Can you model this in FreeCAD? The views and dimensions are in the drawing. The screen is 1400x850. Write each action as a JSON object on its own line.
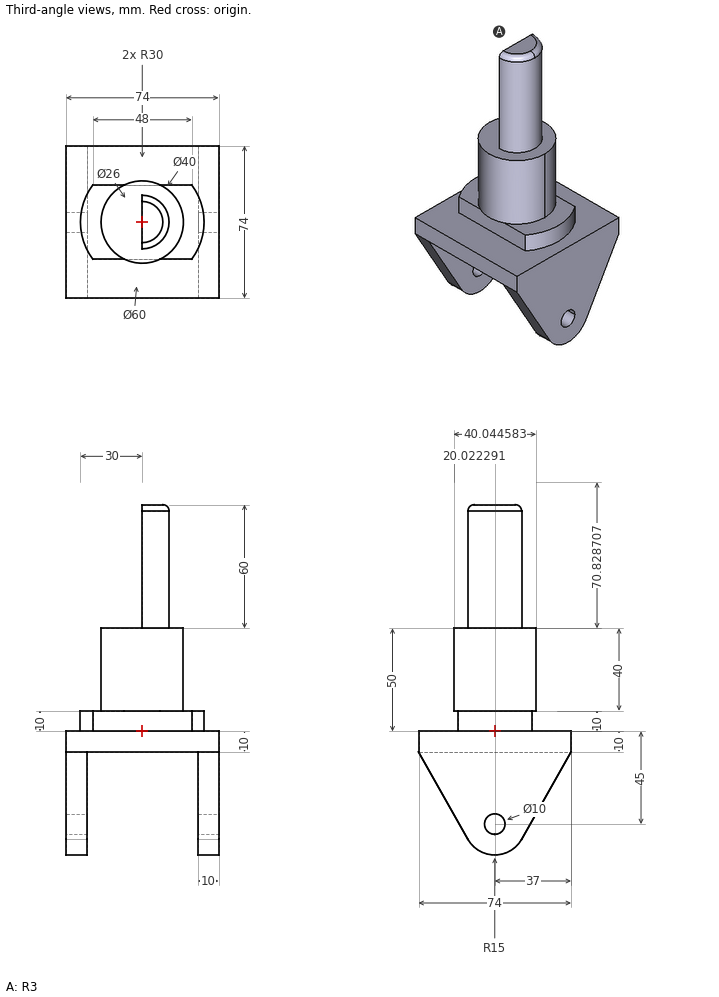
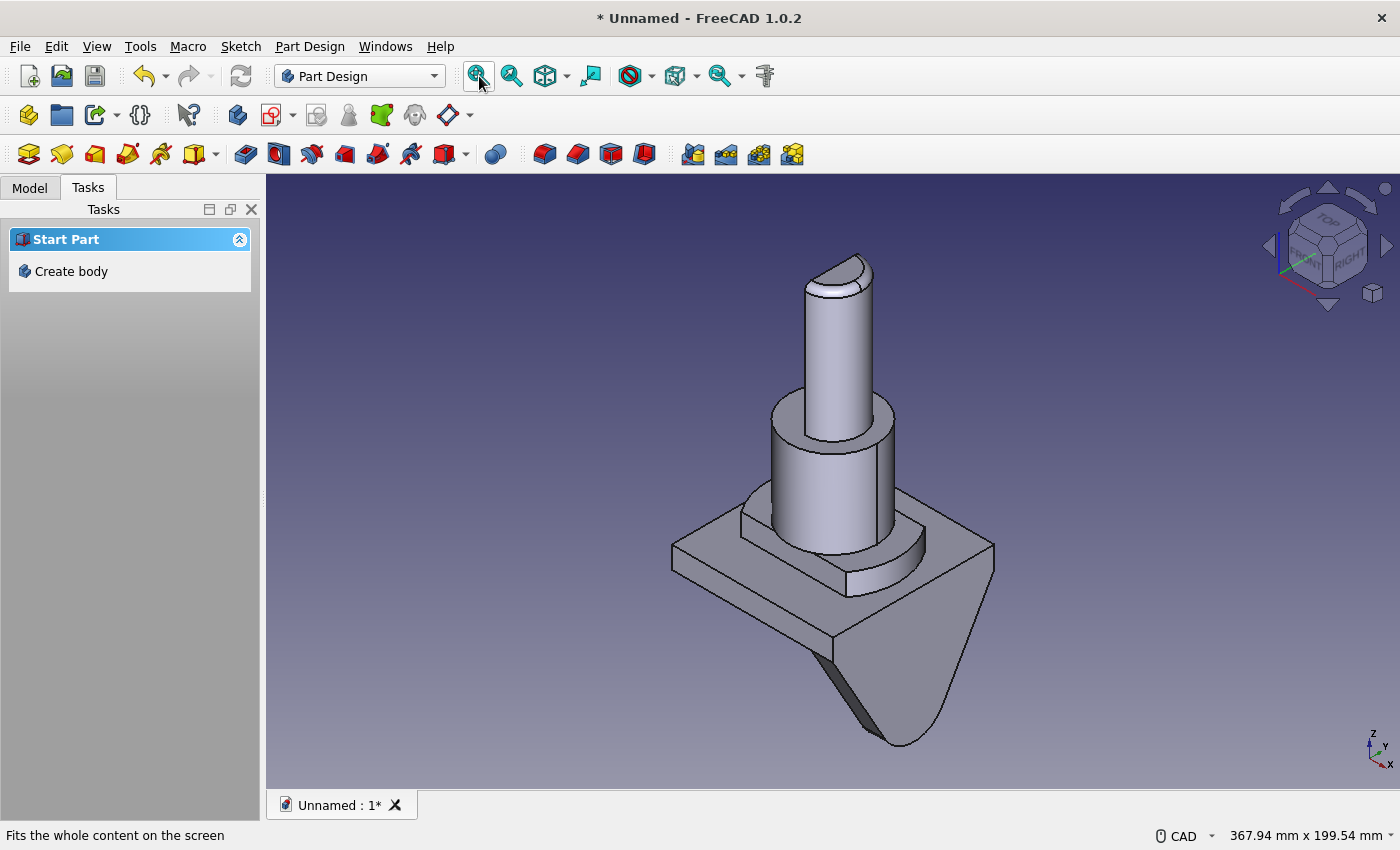
{"action": "left_click", "coordinate": [30, 188]}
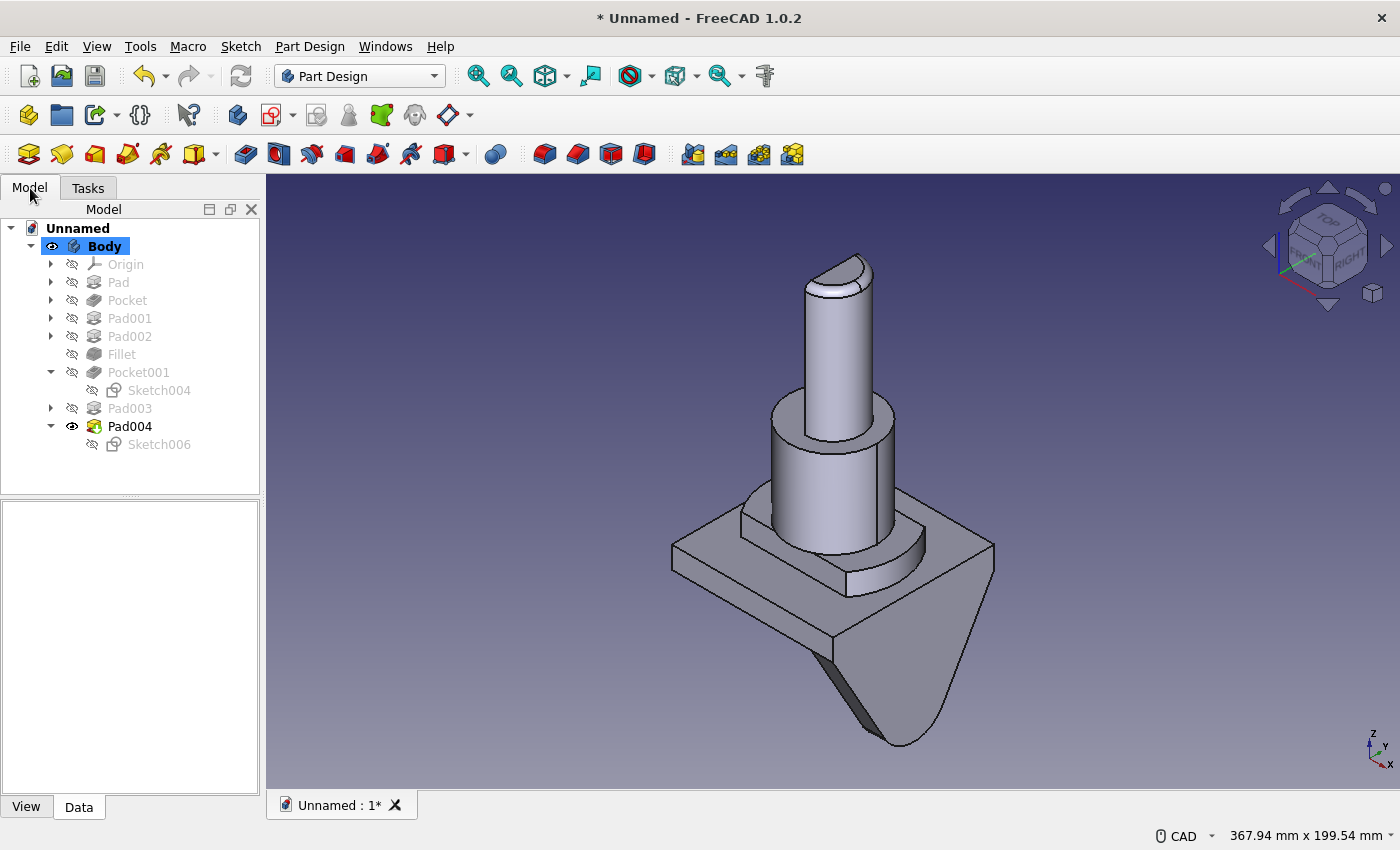
{"action": "left_click", "coordinate": [117, 426]}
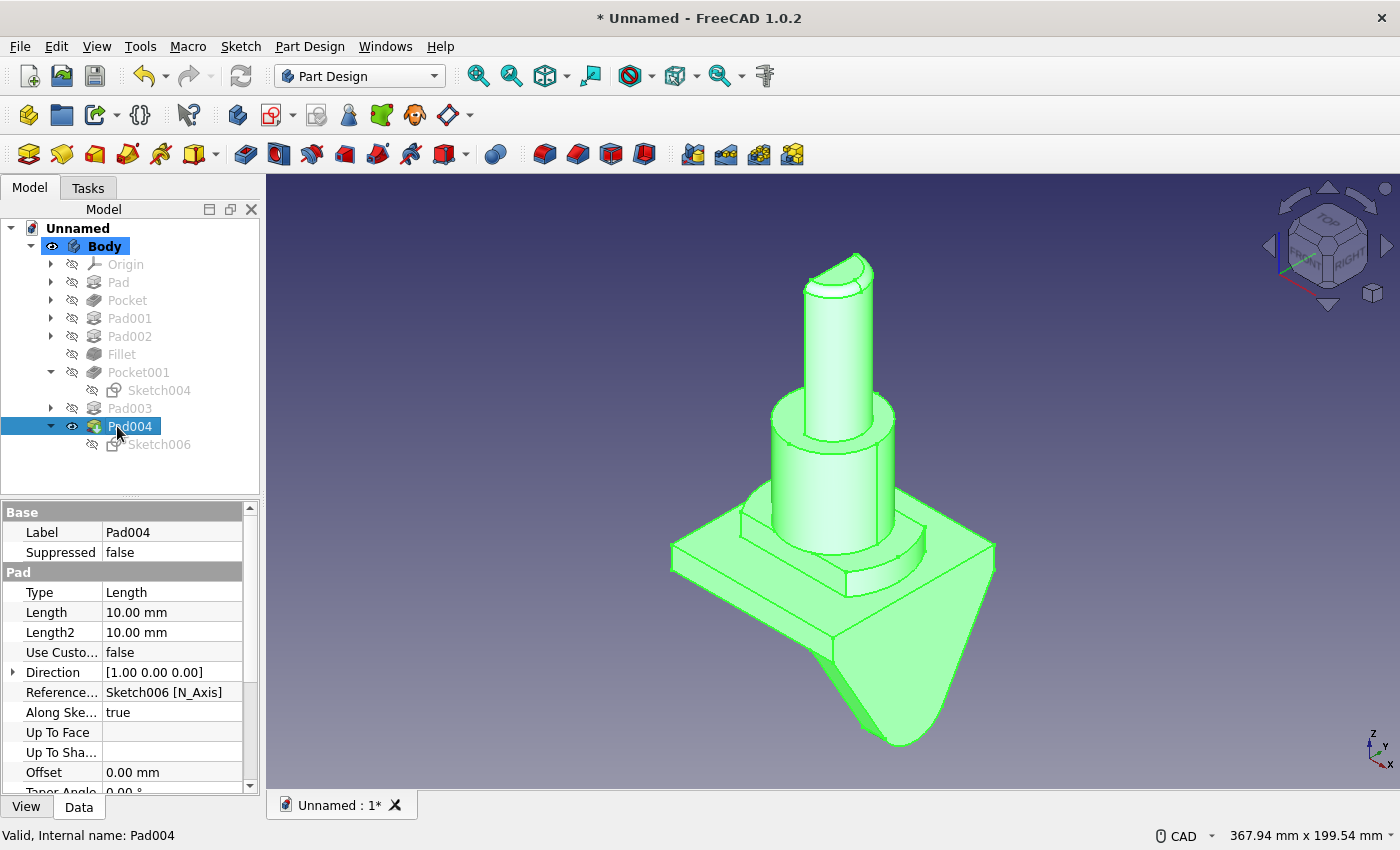
{"action": "left_click", "coordinate": [693, 154]}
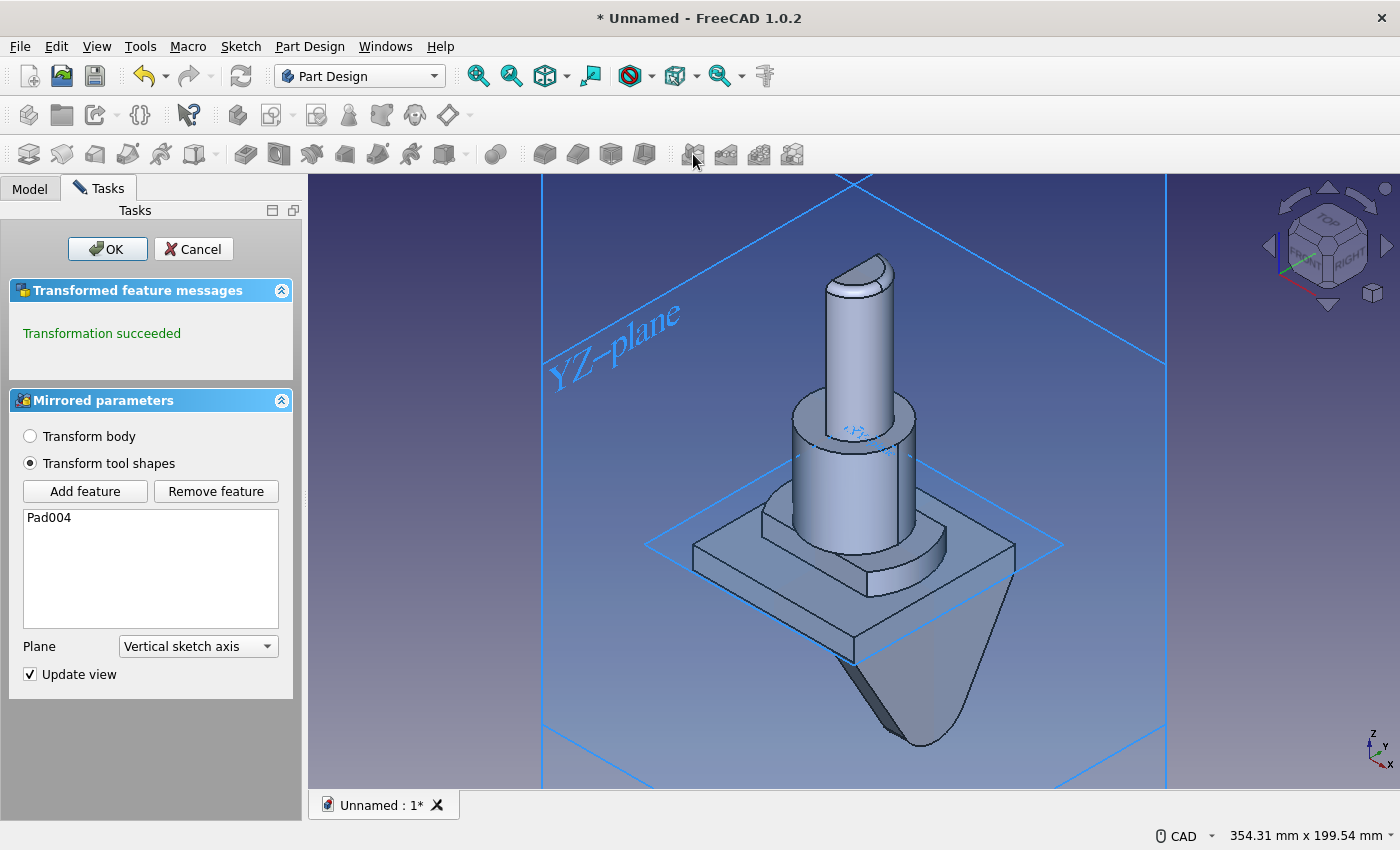
{"action": "left_click", "coordinate": [199, 646]}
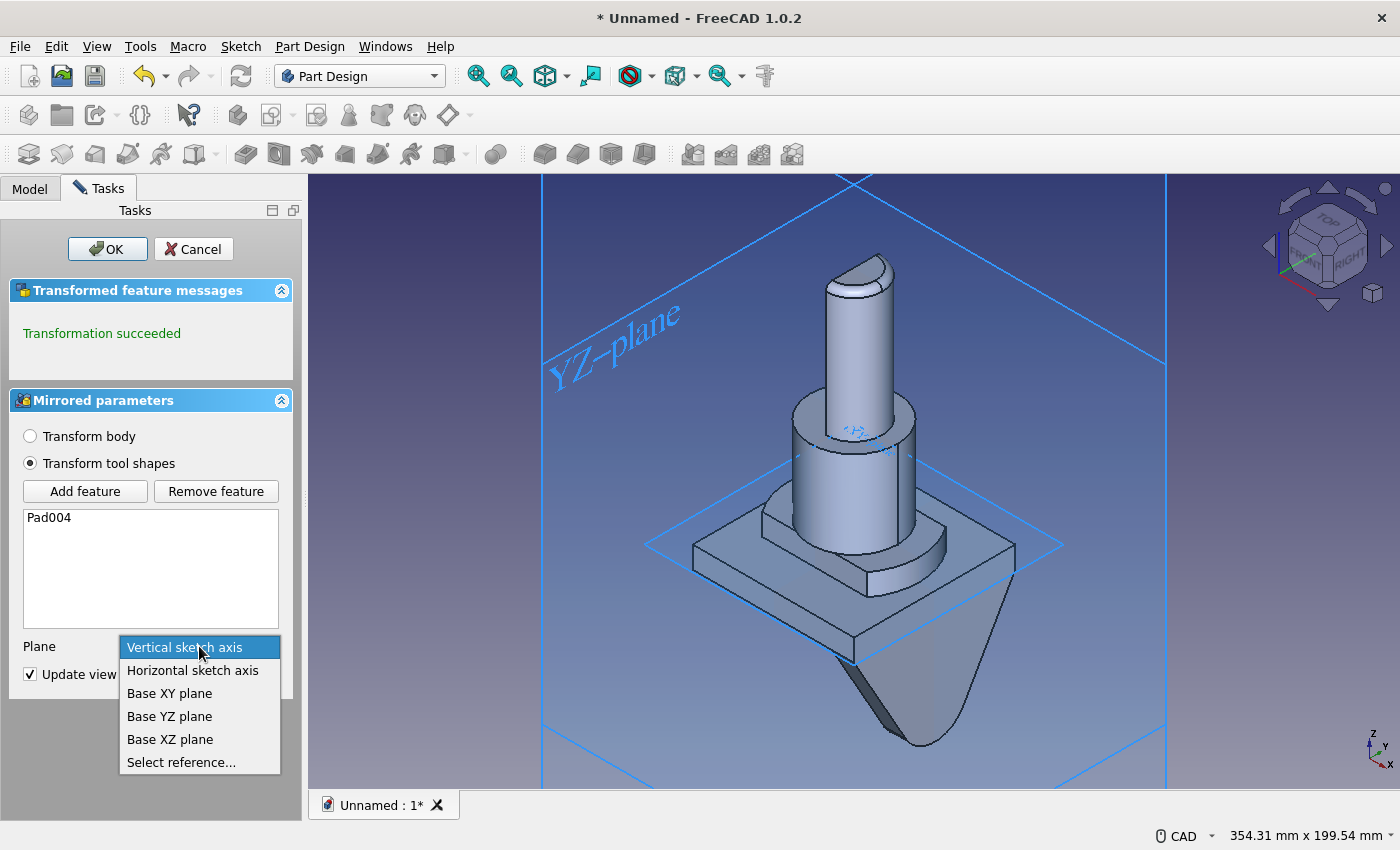
{"action": "left_click", "coordinate": [198, 716]}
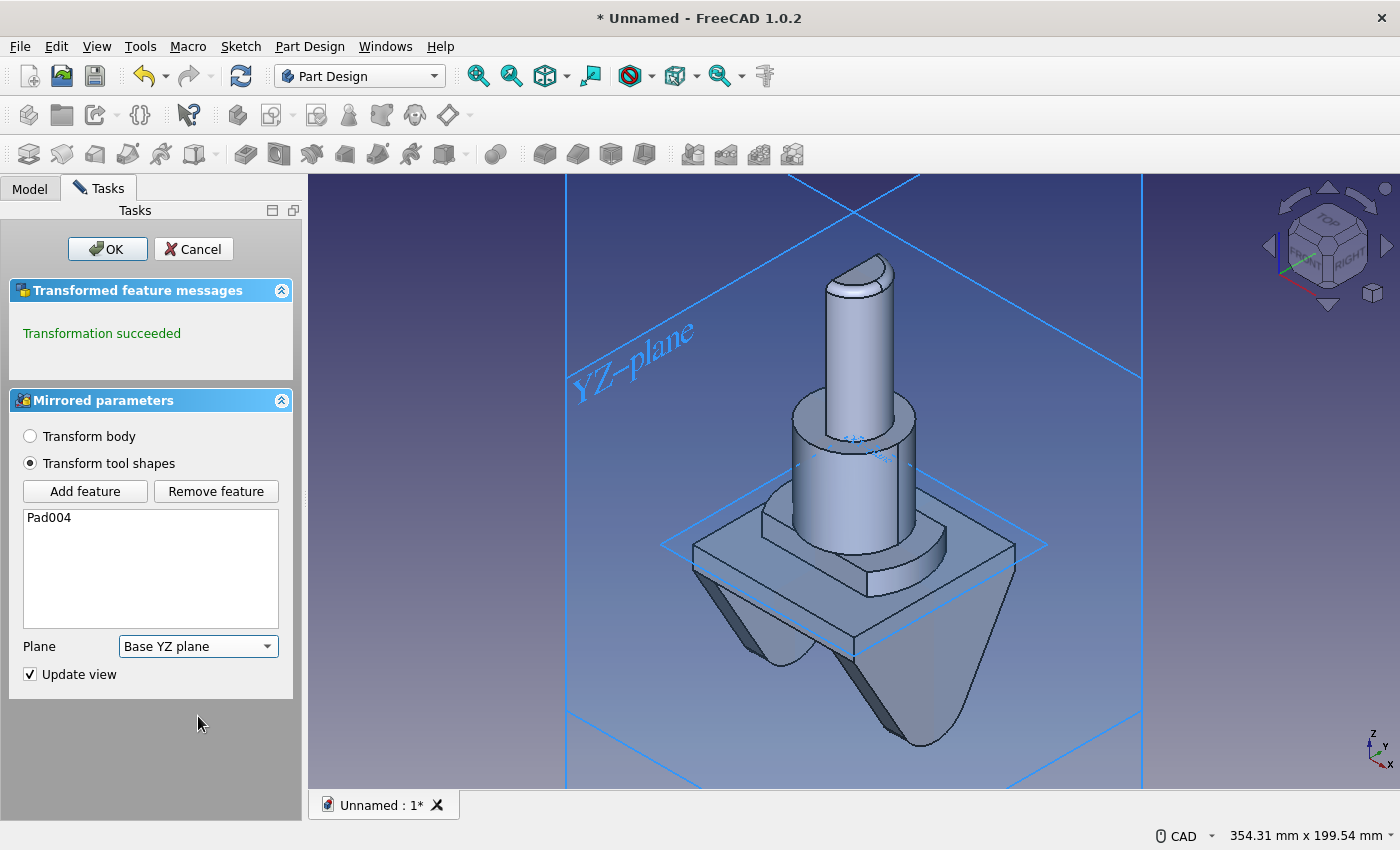
{"action": "left_click", "coordinate": [108, 249]}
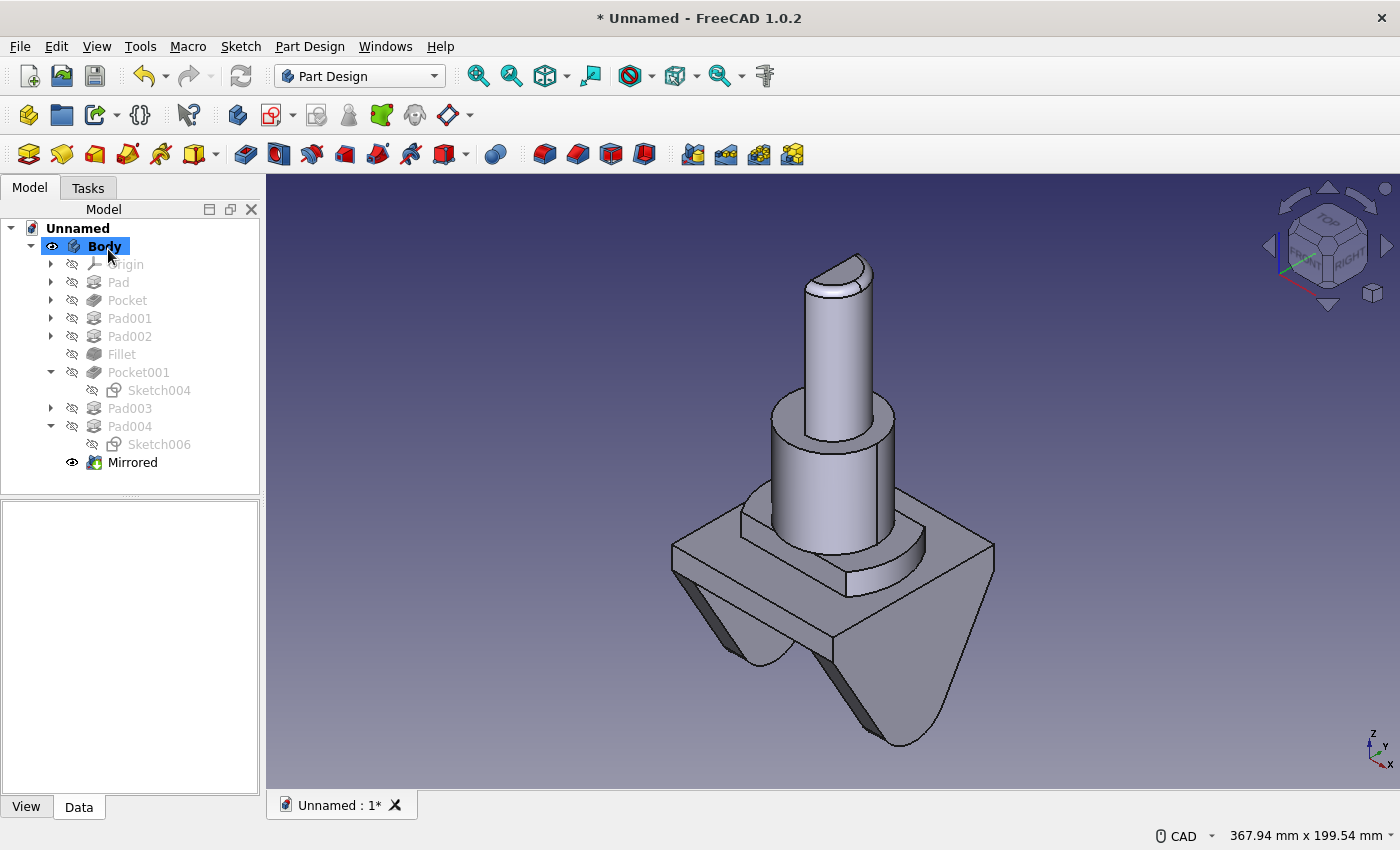
{"action": "left_click", "coordinate": [914, 666]}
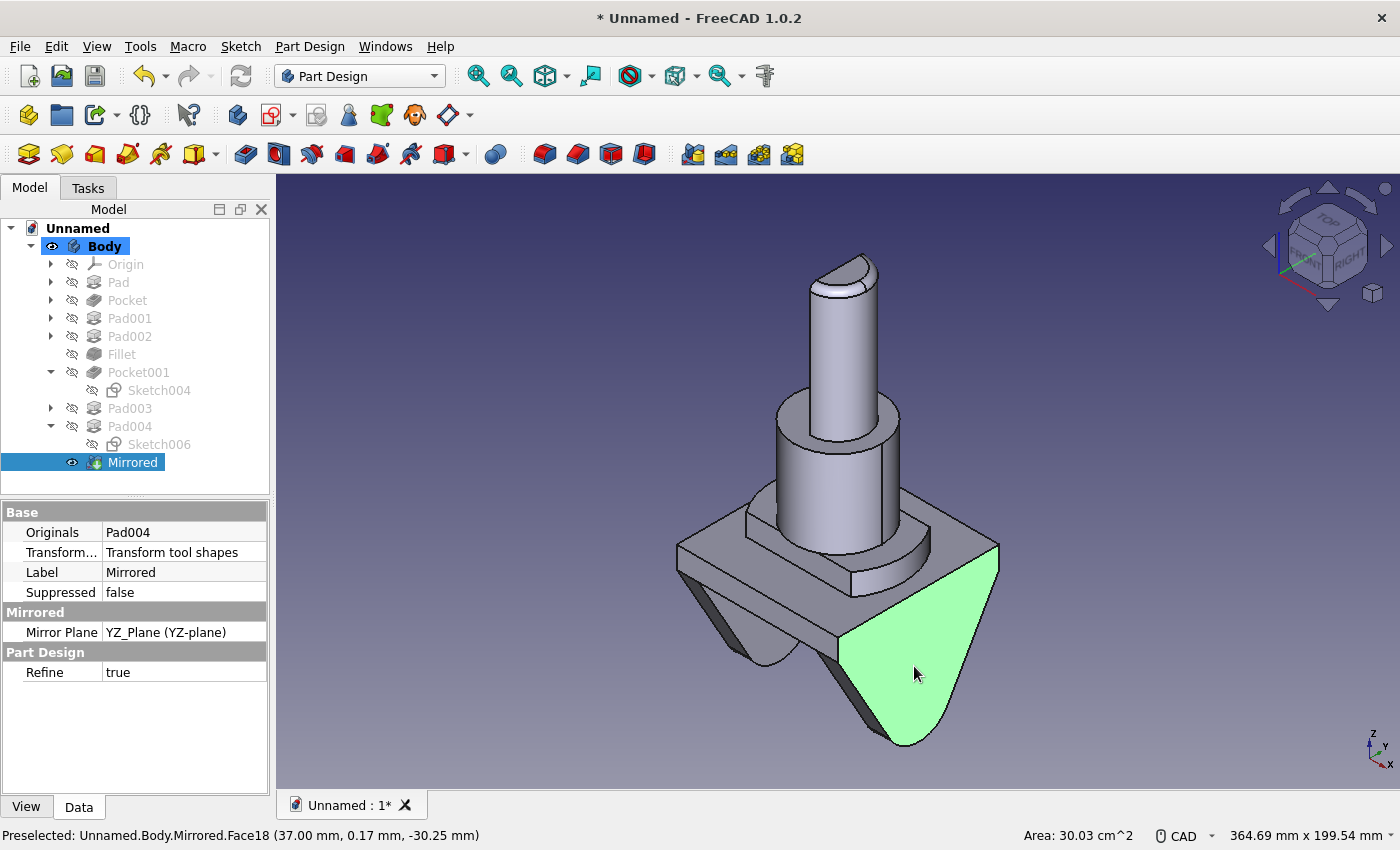
{"action": "left_click", "coordinate": [270, 116]}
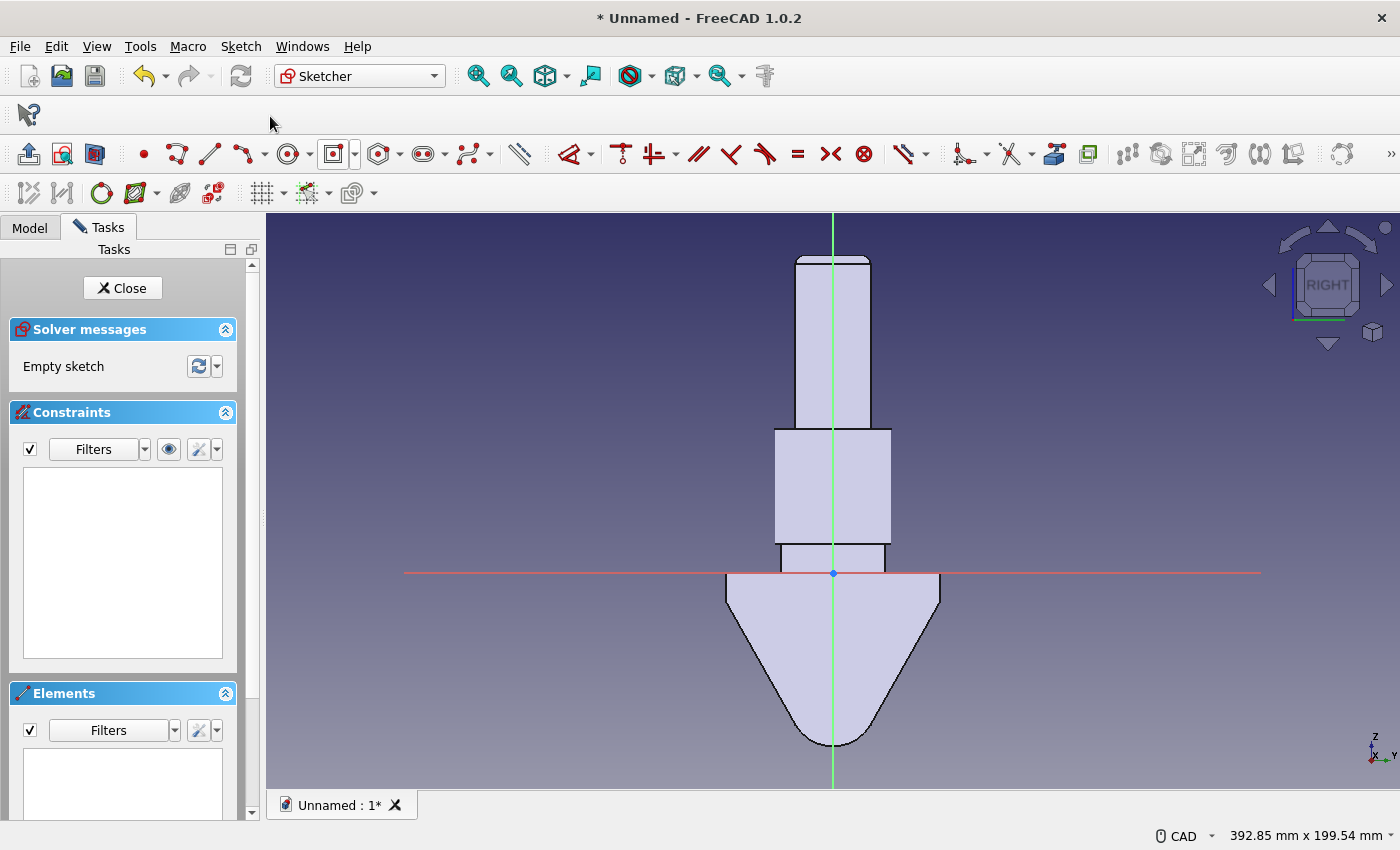
{"action": "scroll", "coordinate": [838, 719], "scroll_direction": "up", "scroll_amount": 13}